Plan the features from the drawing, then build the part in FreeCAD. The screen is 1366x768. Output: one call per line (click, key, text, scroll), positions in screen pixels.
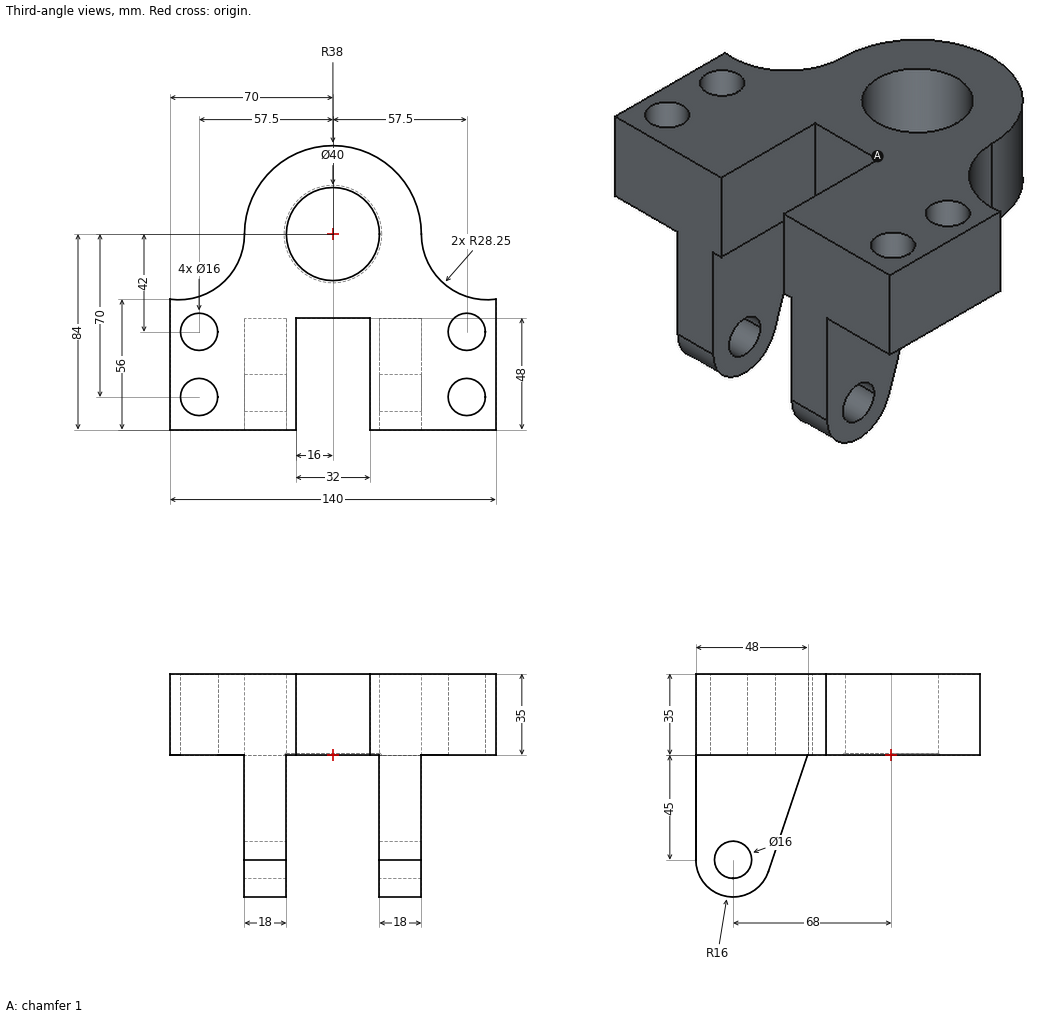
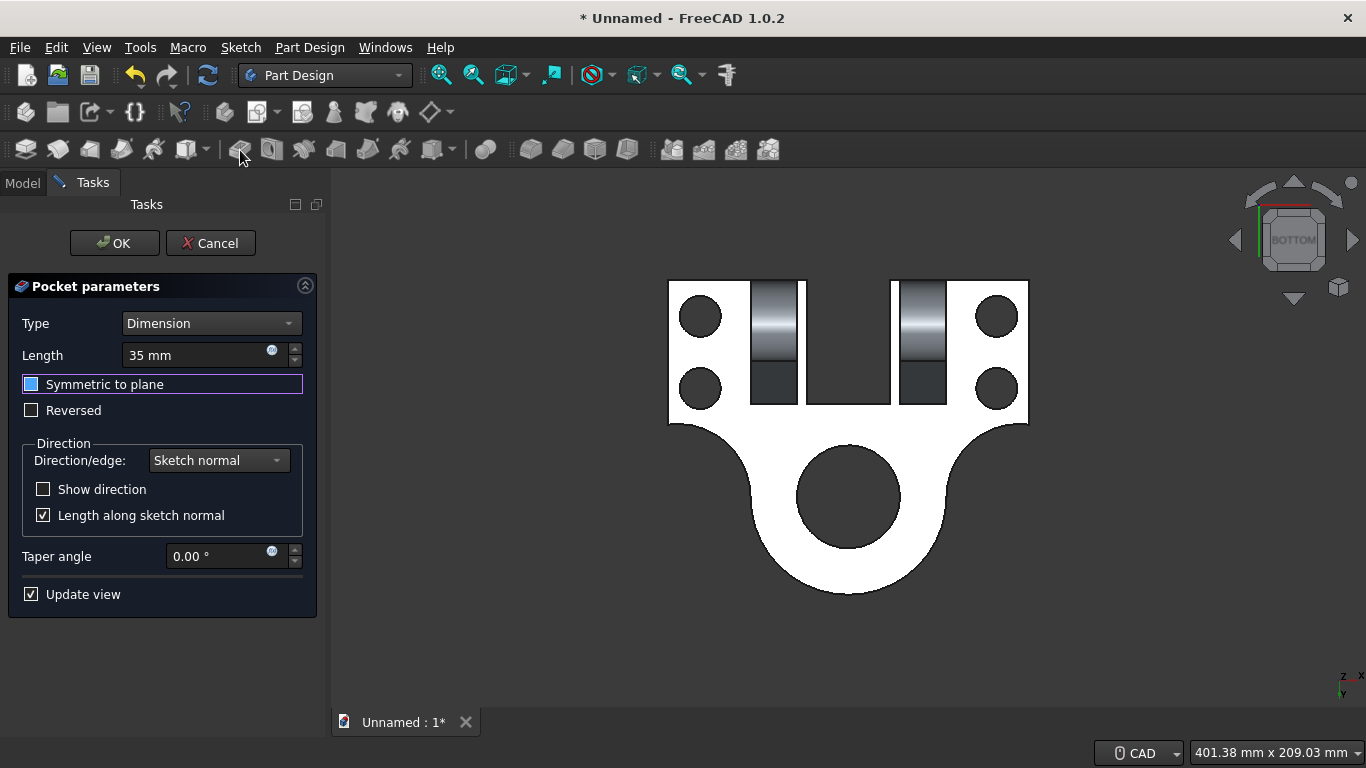
click(115, 243)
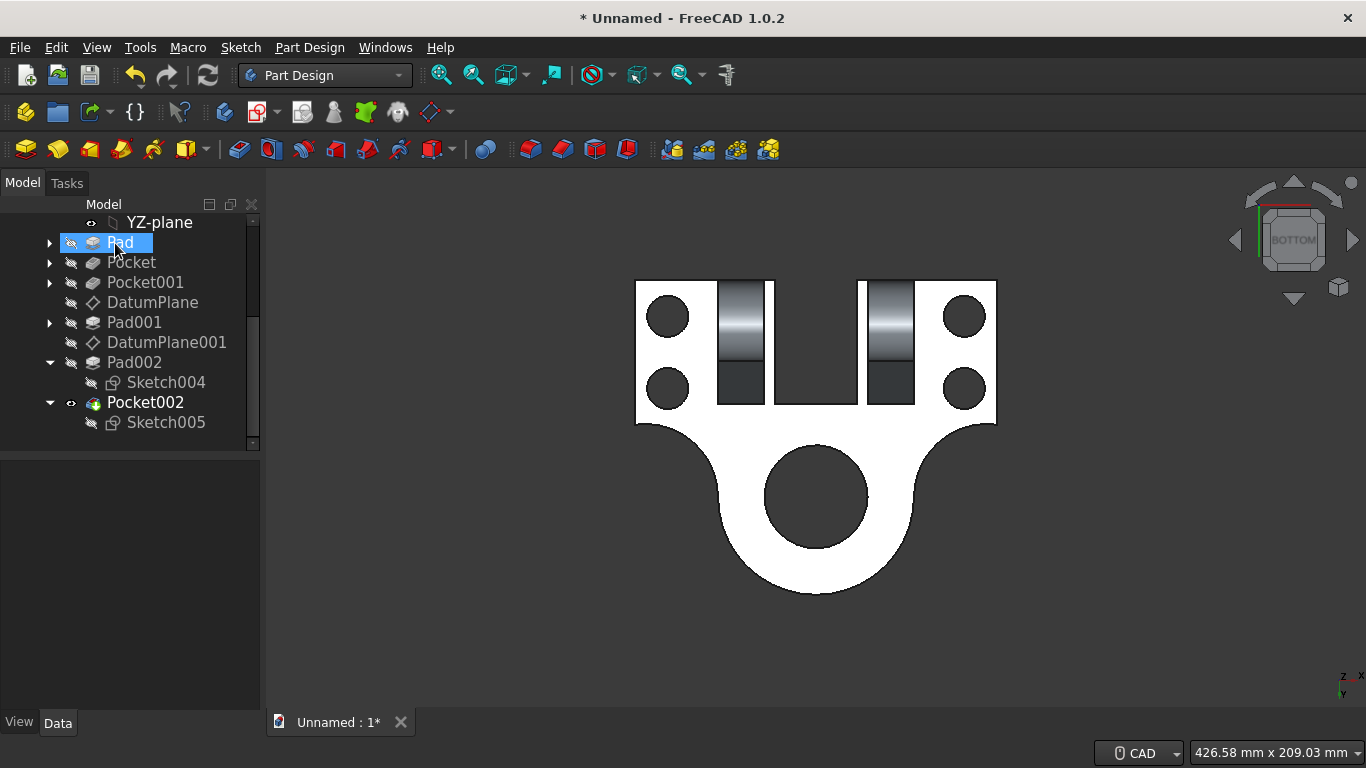
click(774, 465)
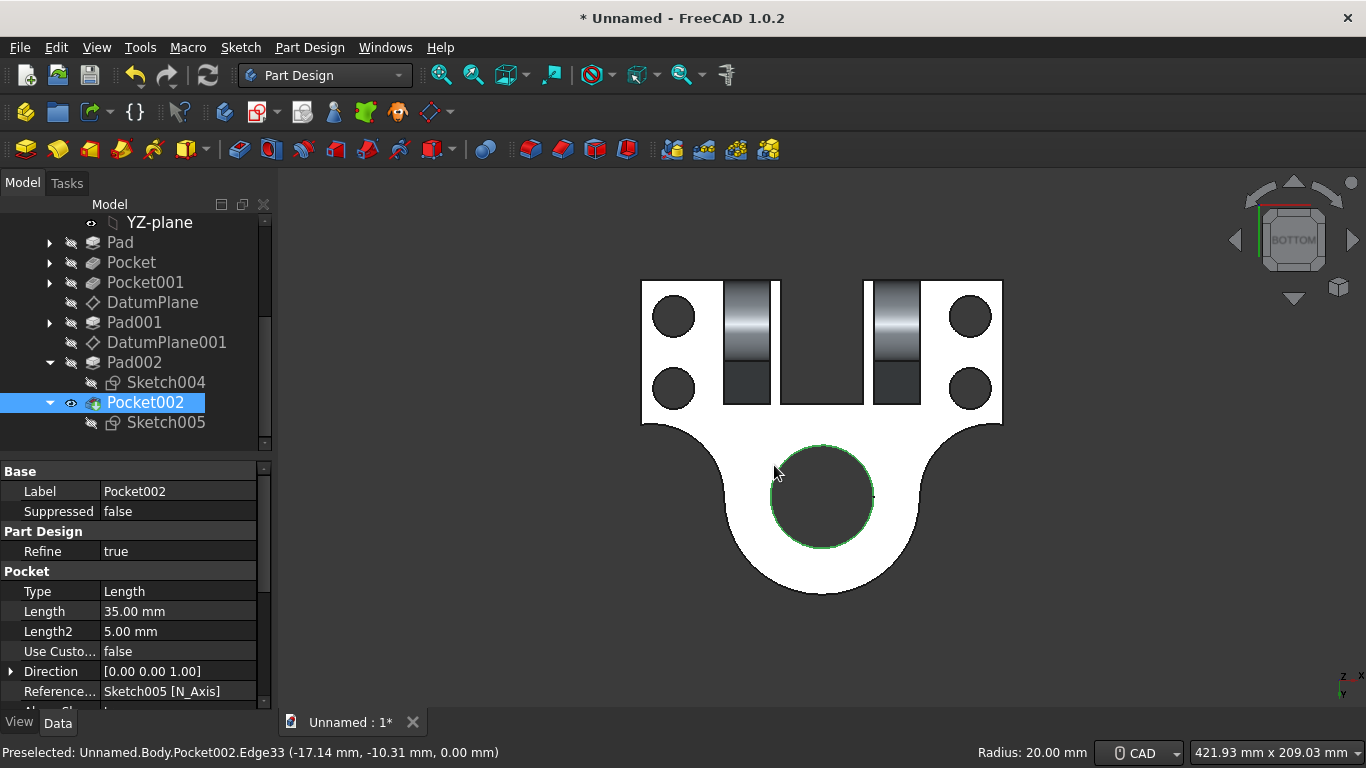
click(564, 150)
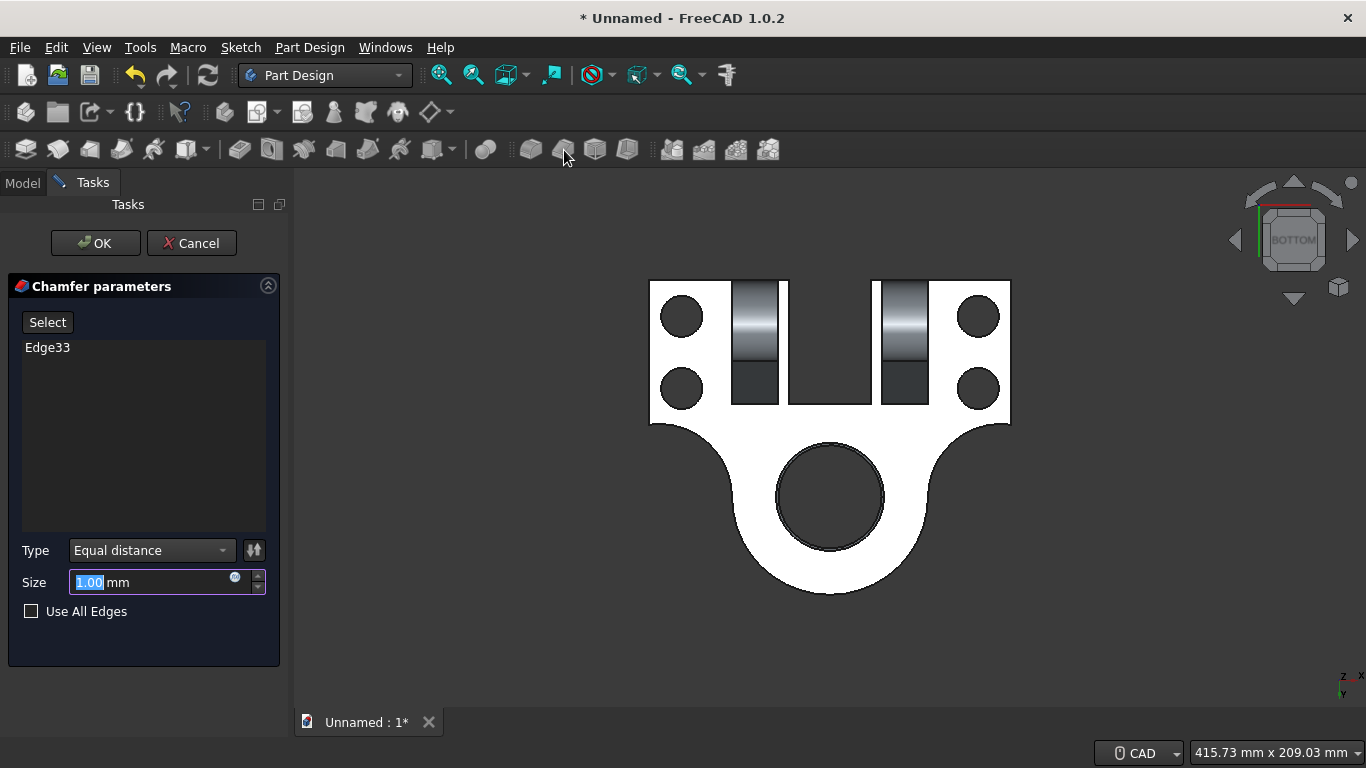
text(1)
key(Tab)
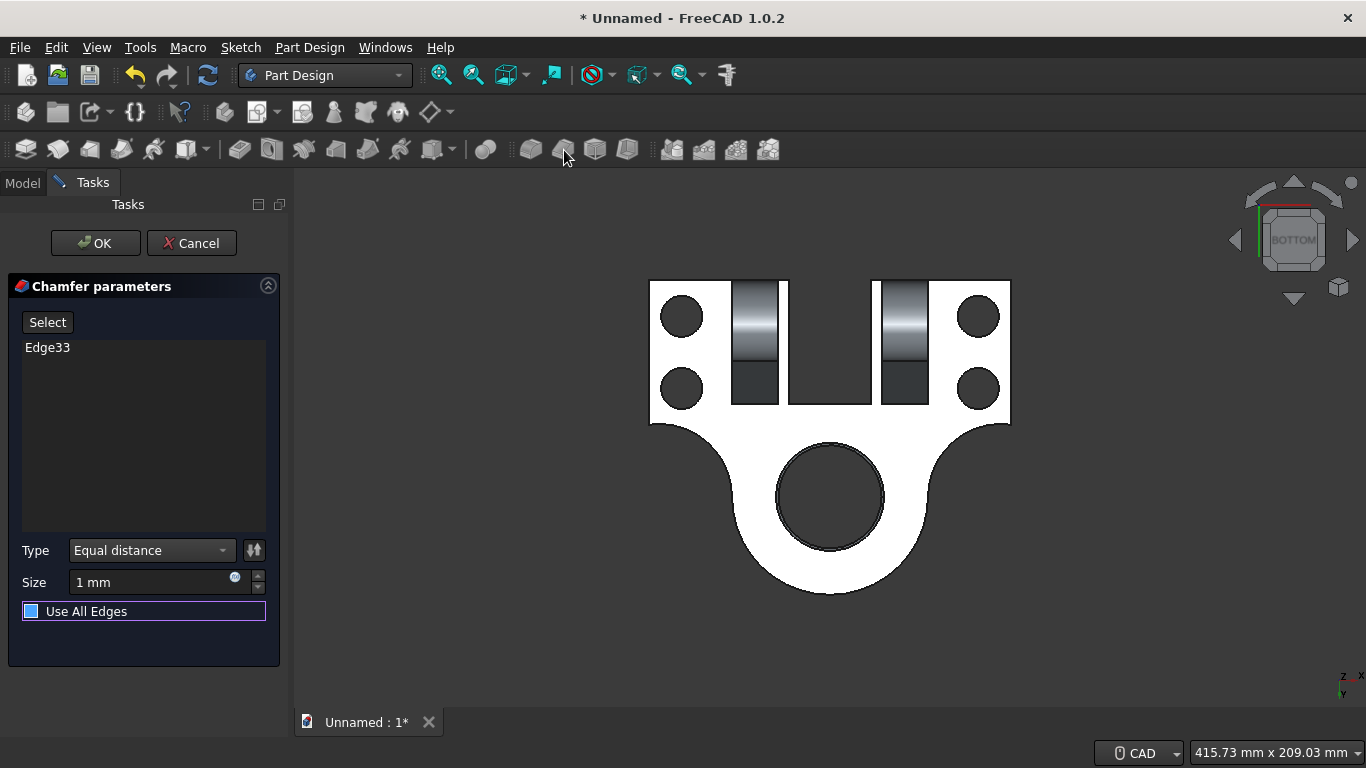
click(96, 243)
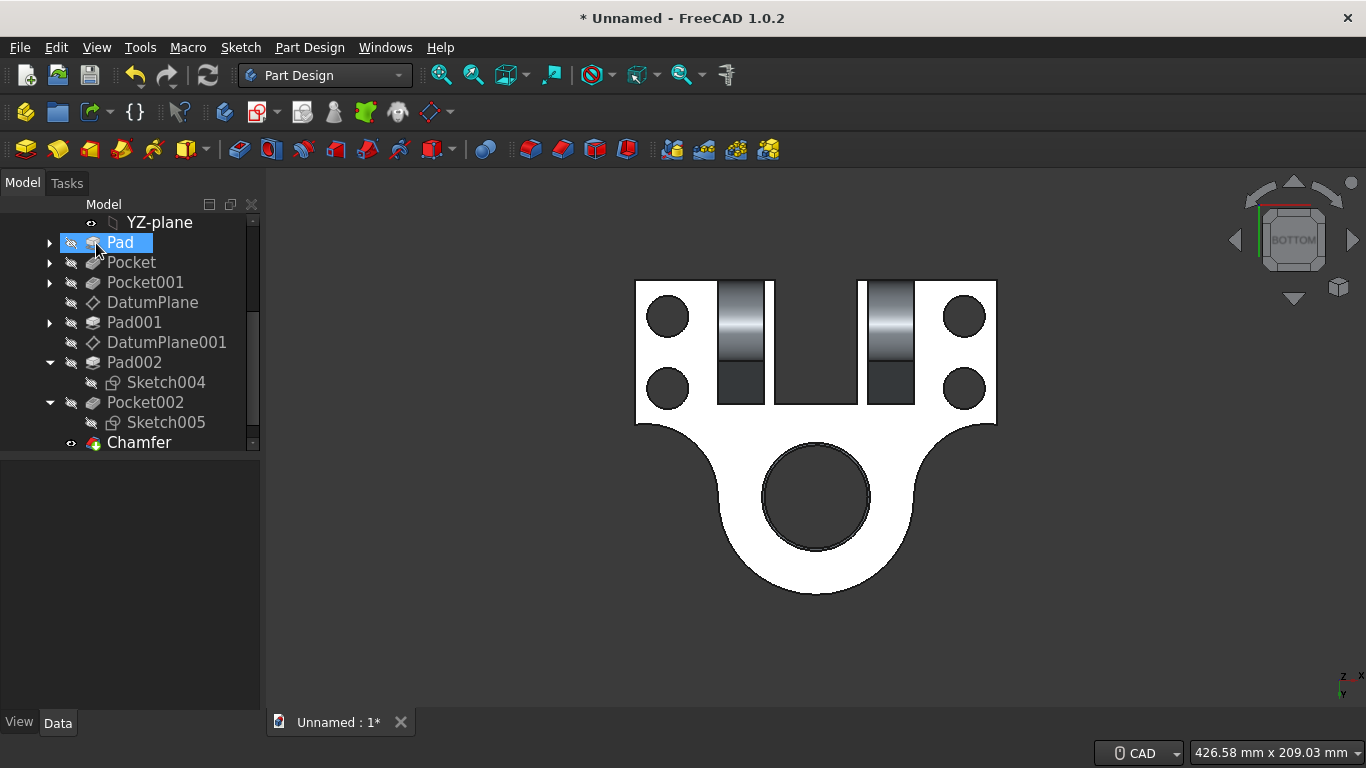
key(0)